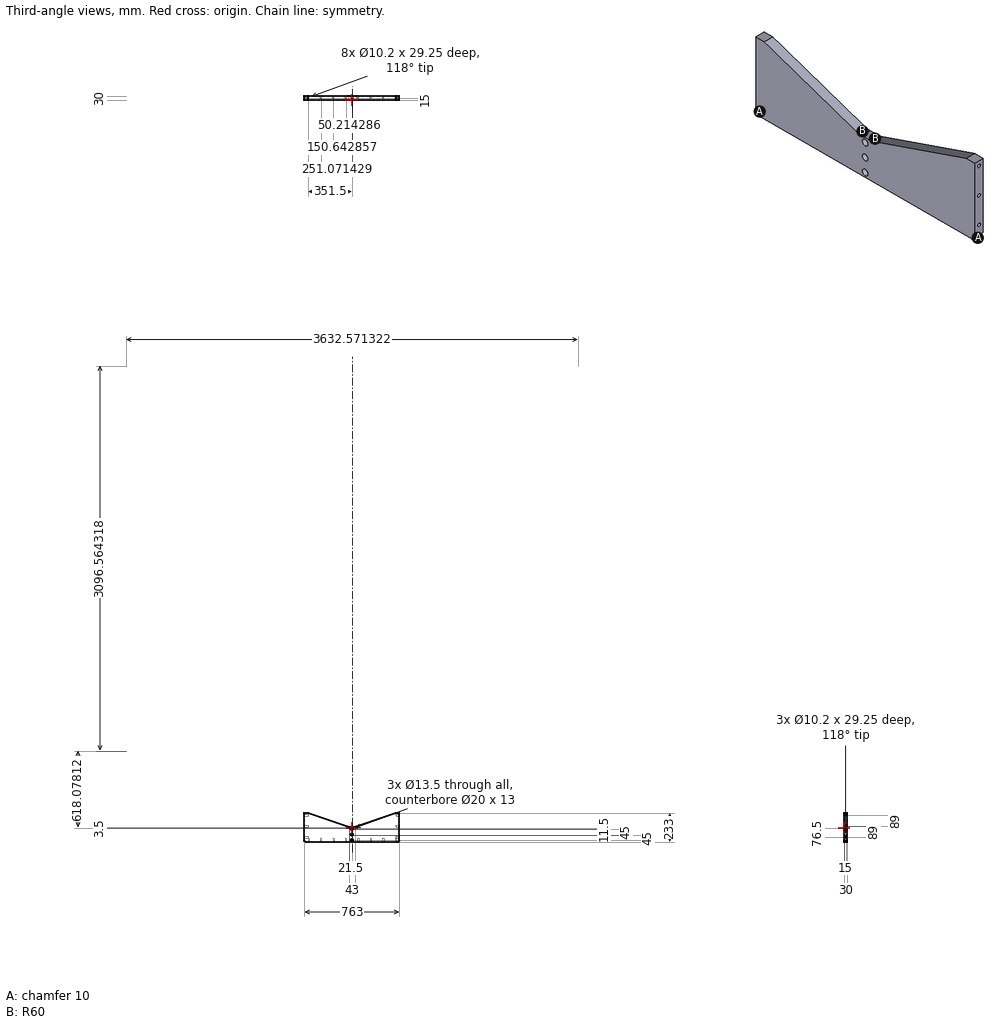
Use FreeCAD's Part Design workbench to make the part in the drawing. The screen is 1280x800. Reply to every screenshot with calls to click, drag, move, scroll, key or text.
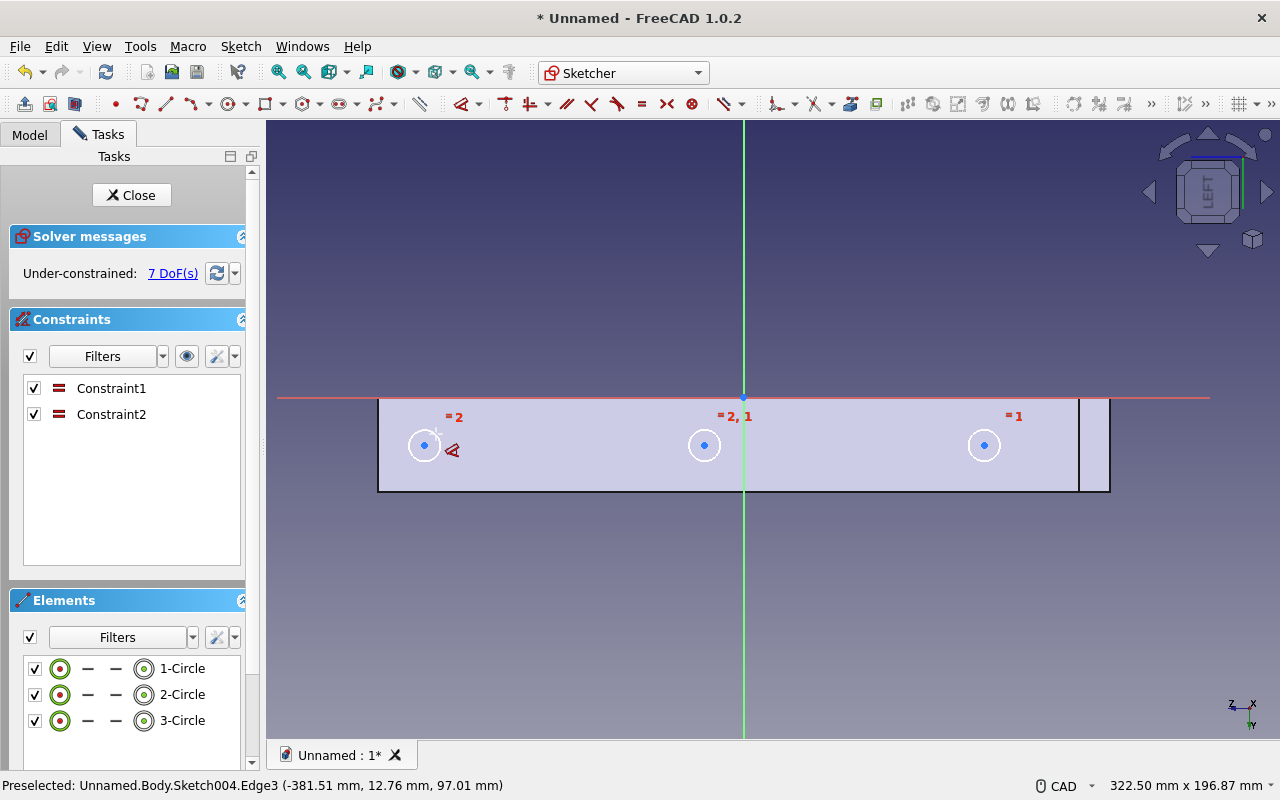
scroll(995, 434, up, 2)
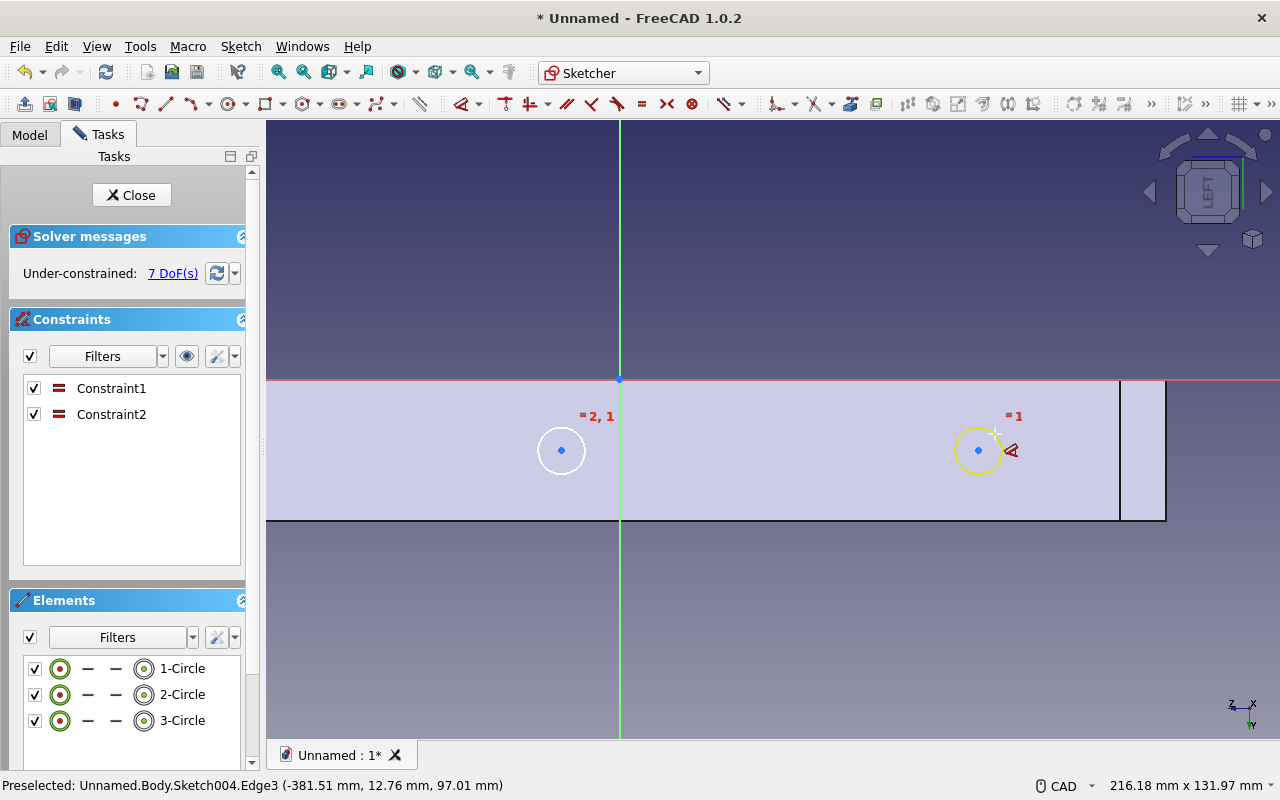
click(995, 434)
click(1017, 411)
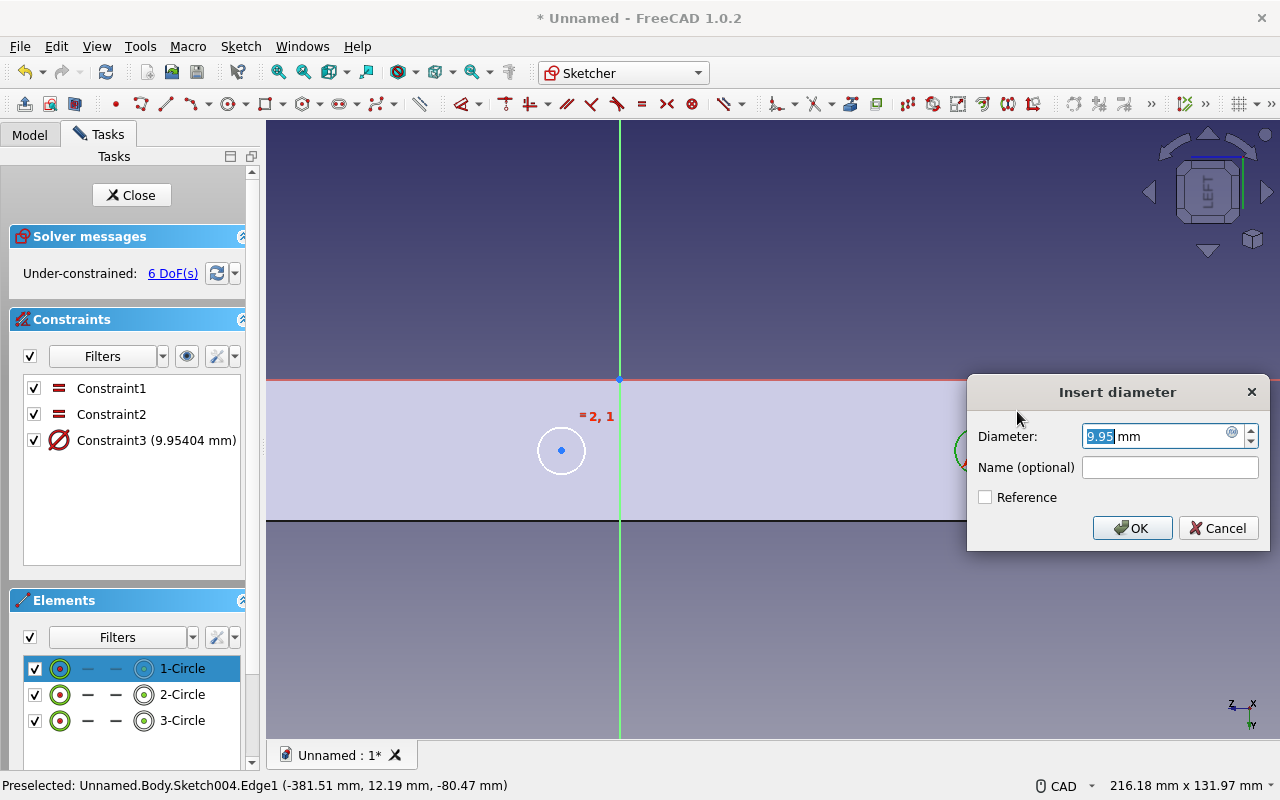
text(10.2)
key(Return)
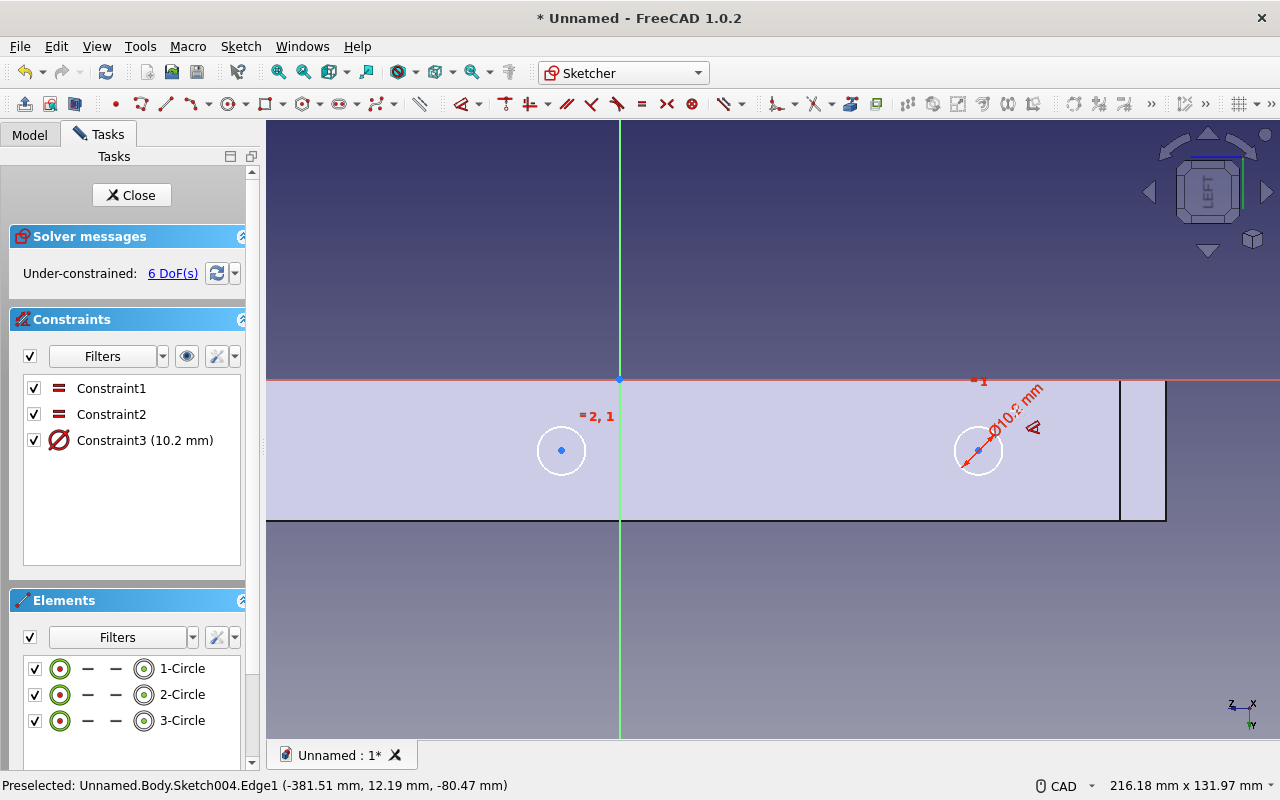
click(979, 451)
click(1013, 432)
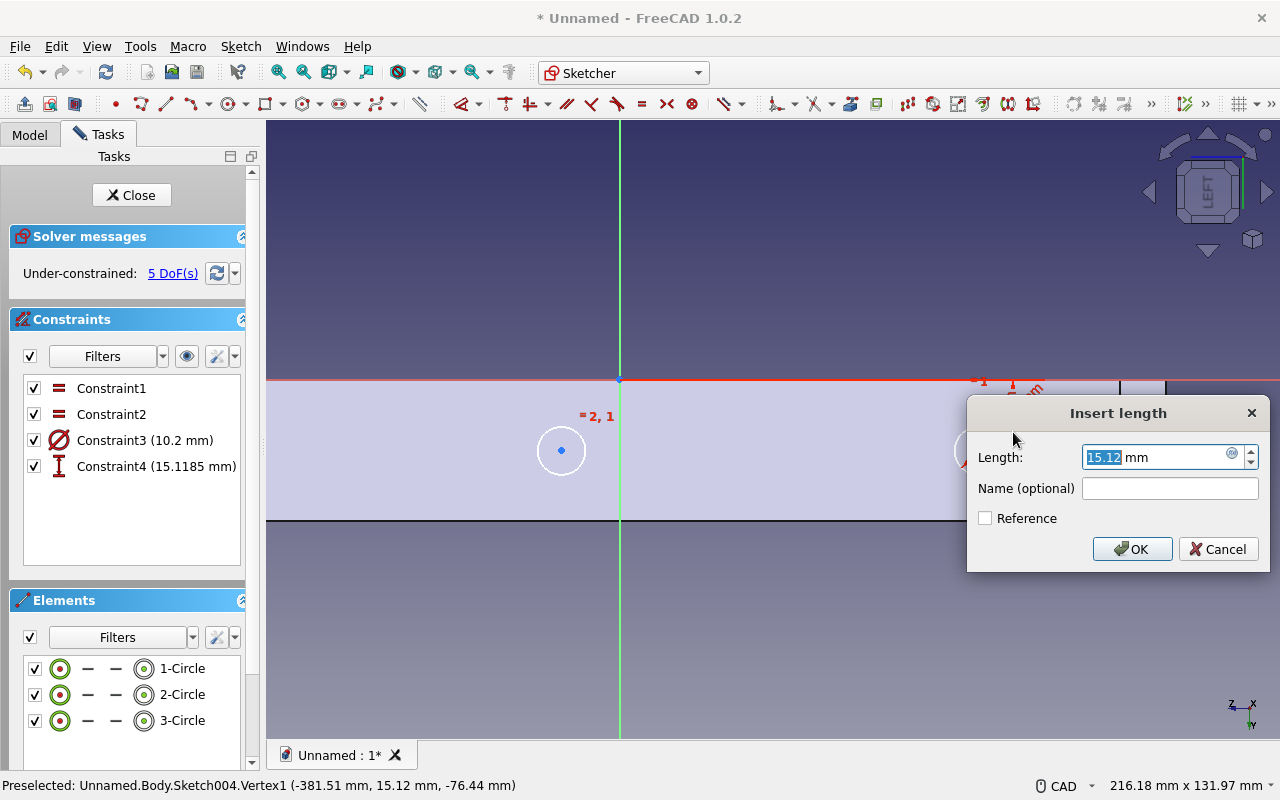
text(15)
key(Return)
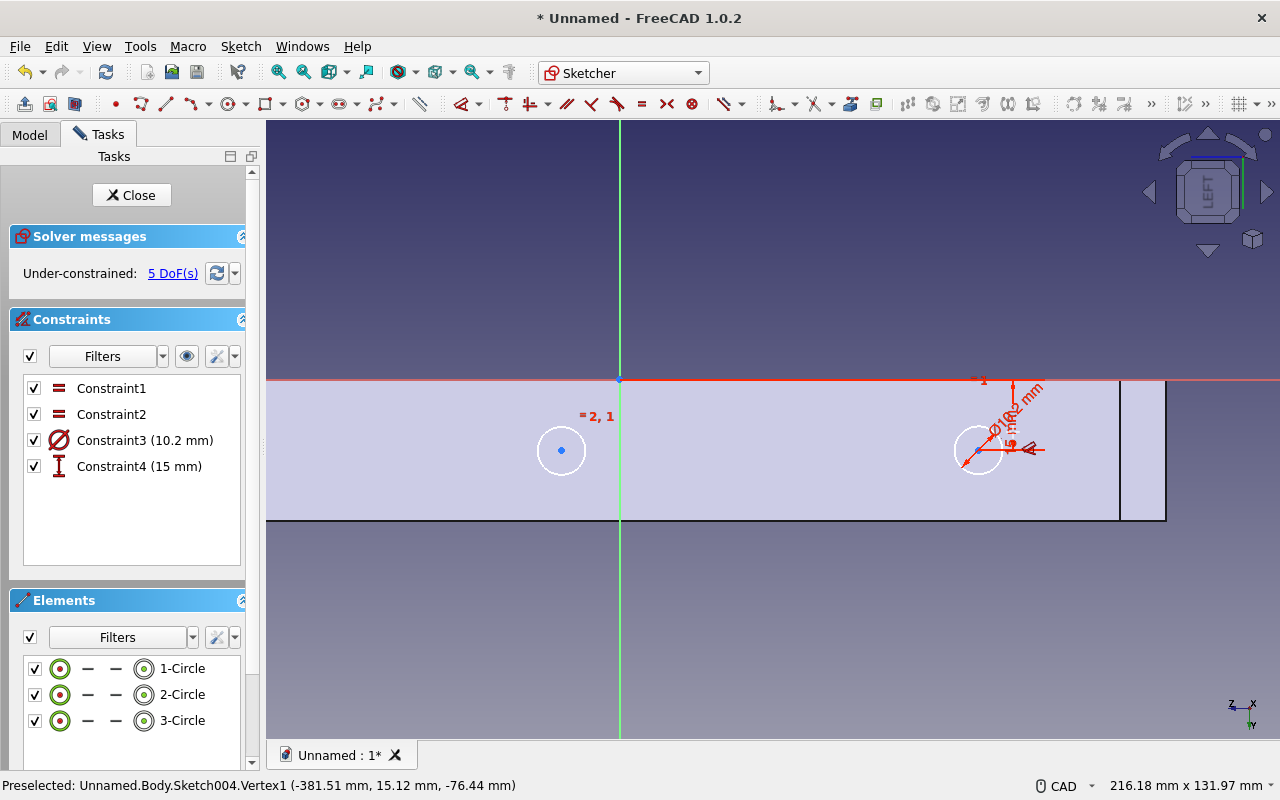
click(562, 451)
click(654, 415)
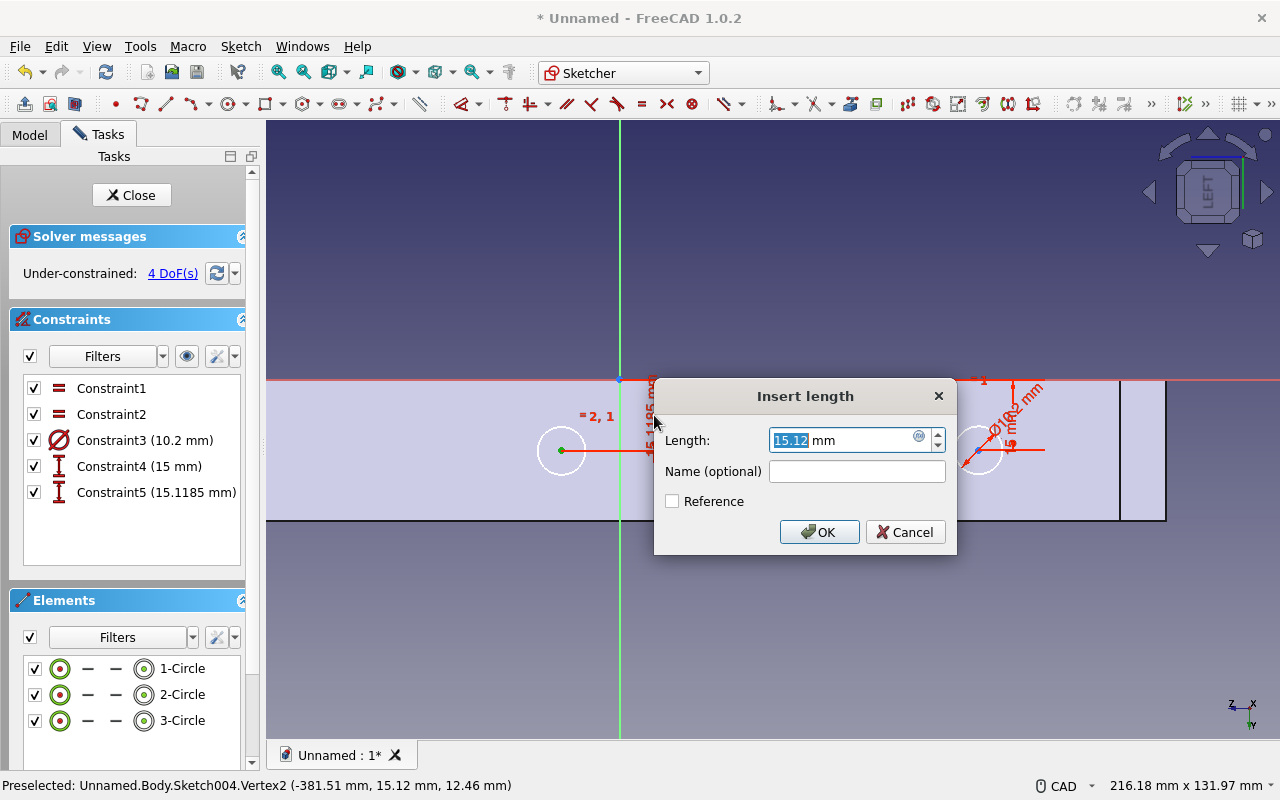
text(15)
key(Return)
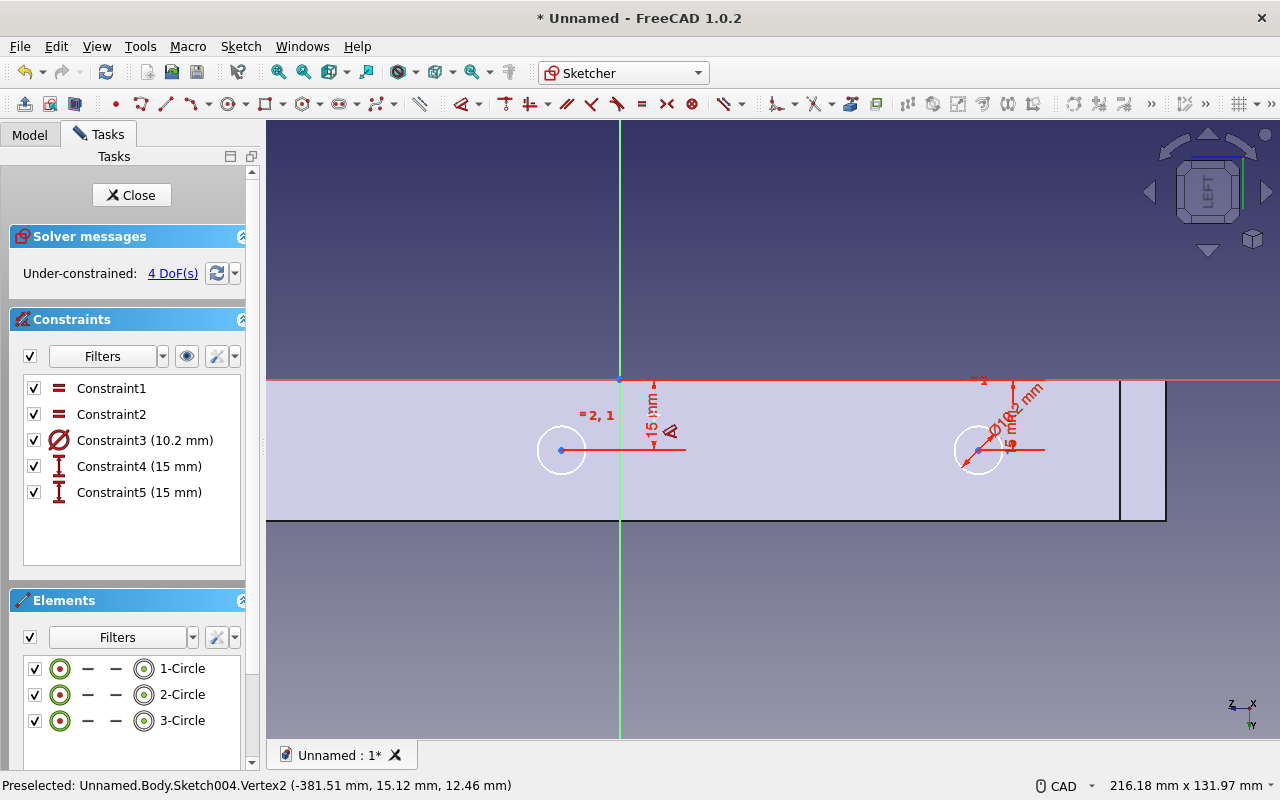
scroll(996, 434, down, 2)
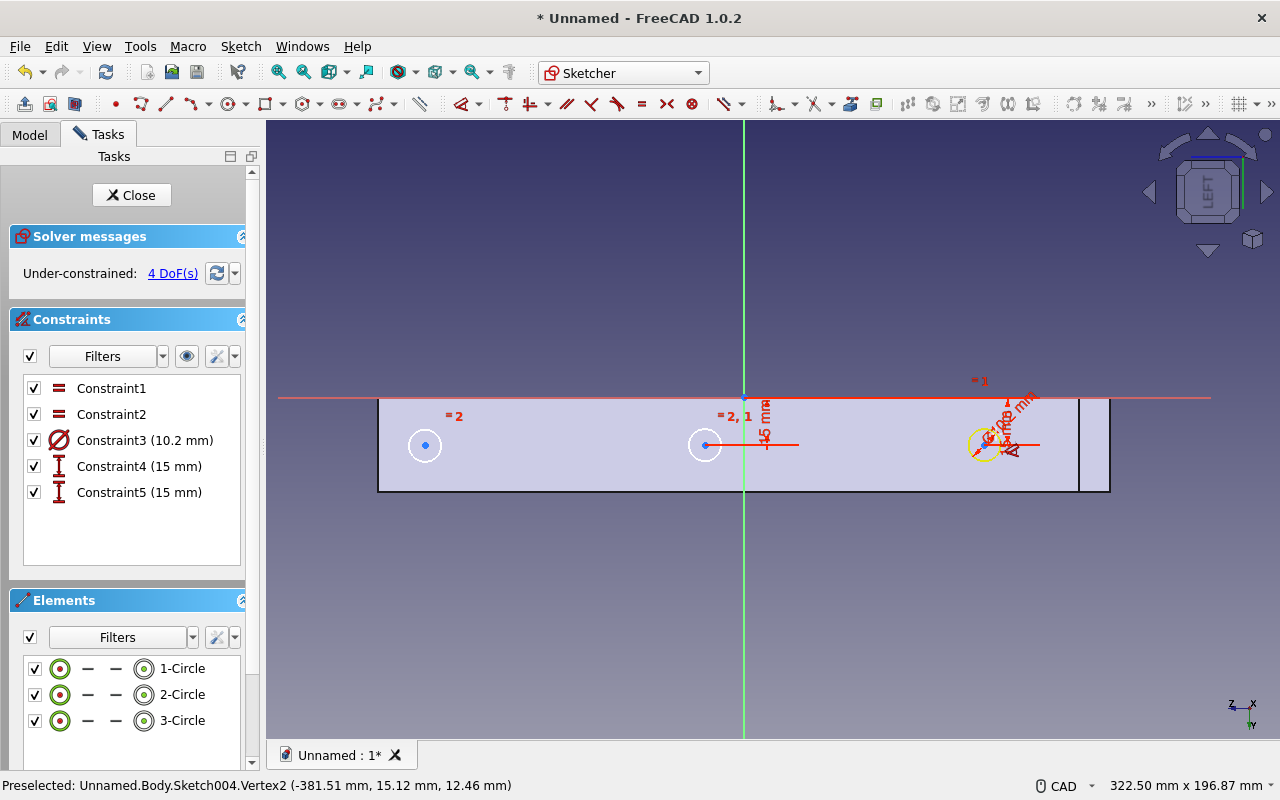
click(425, 446)
click(391, 422)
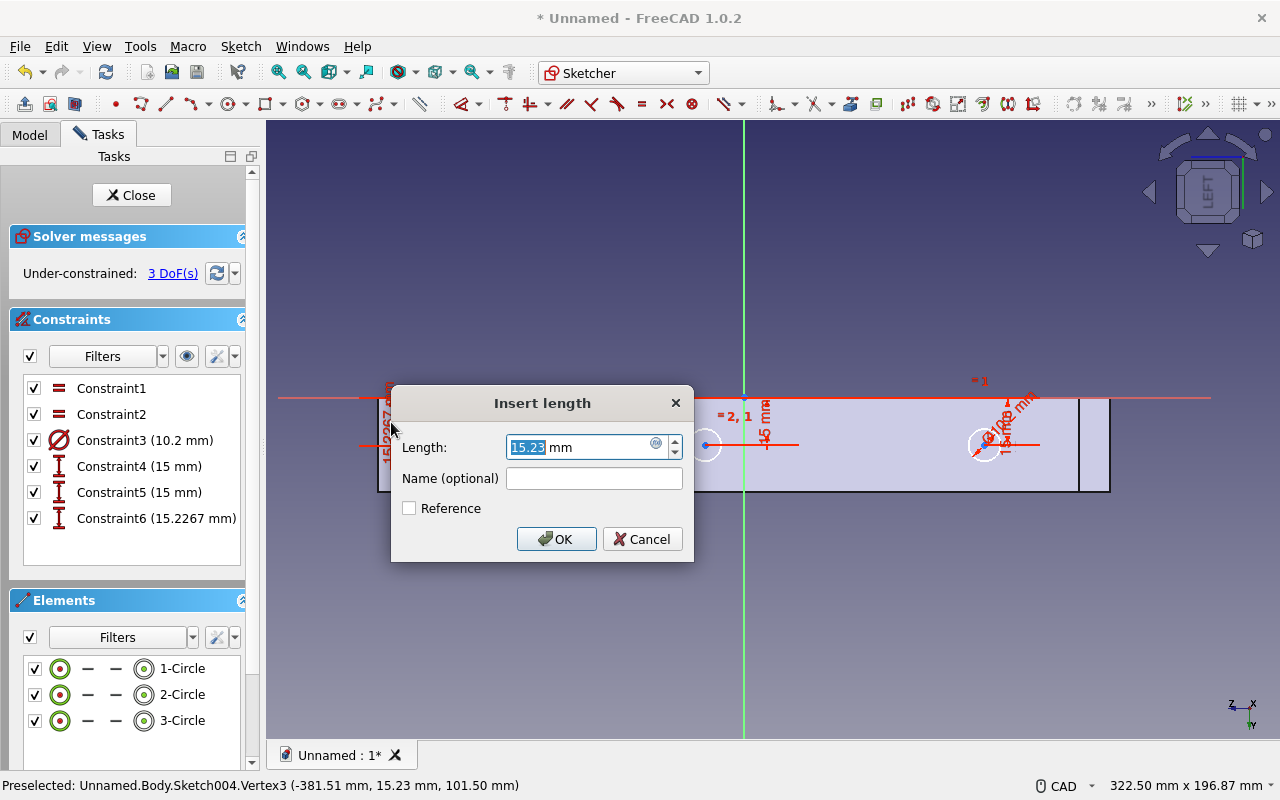
text(15)
key(Return)